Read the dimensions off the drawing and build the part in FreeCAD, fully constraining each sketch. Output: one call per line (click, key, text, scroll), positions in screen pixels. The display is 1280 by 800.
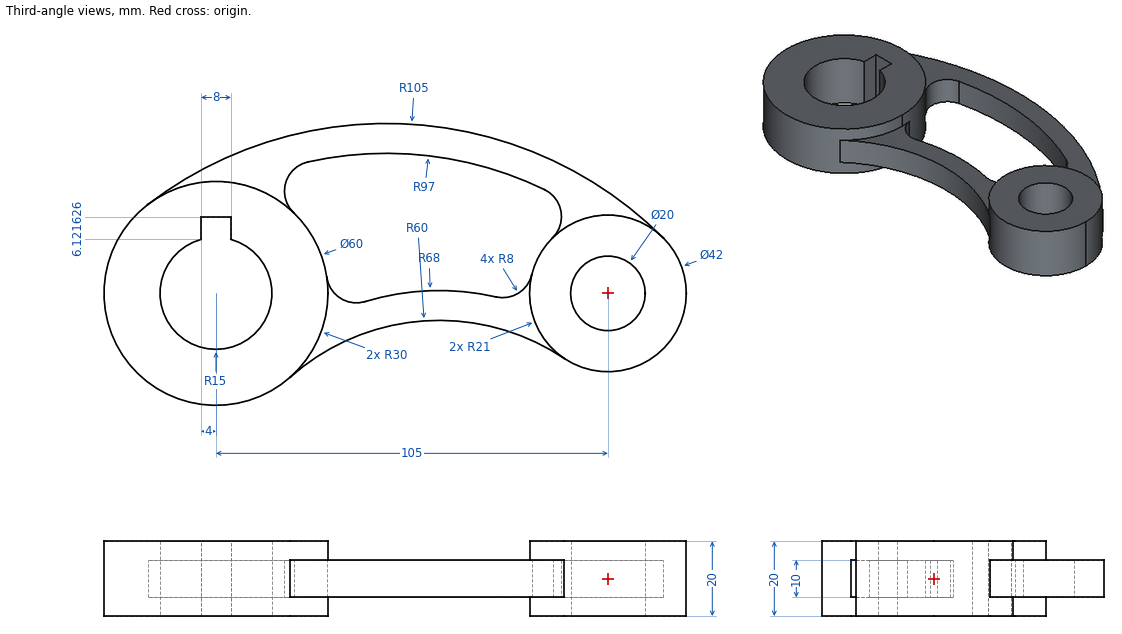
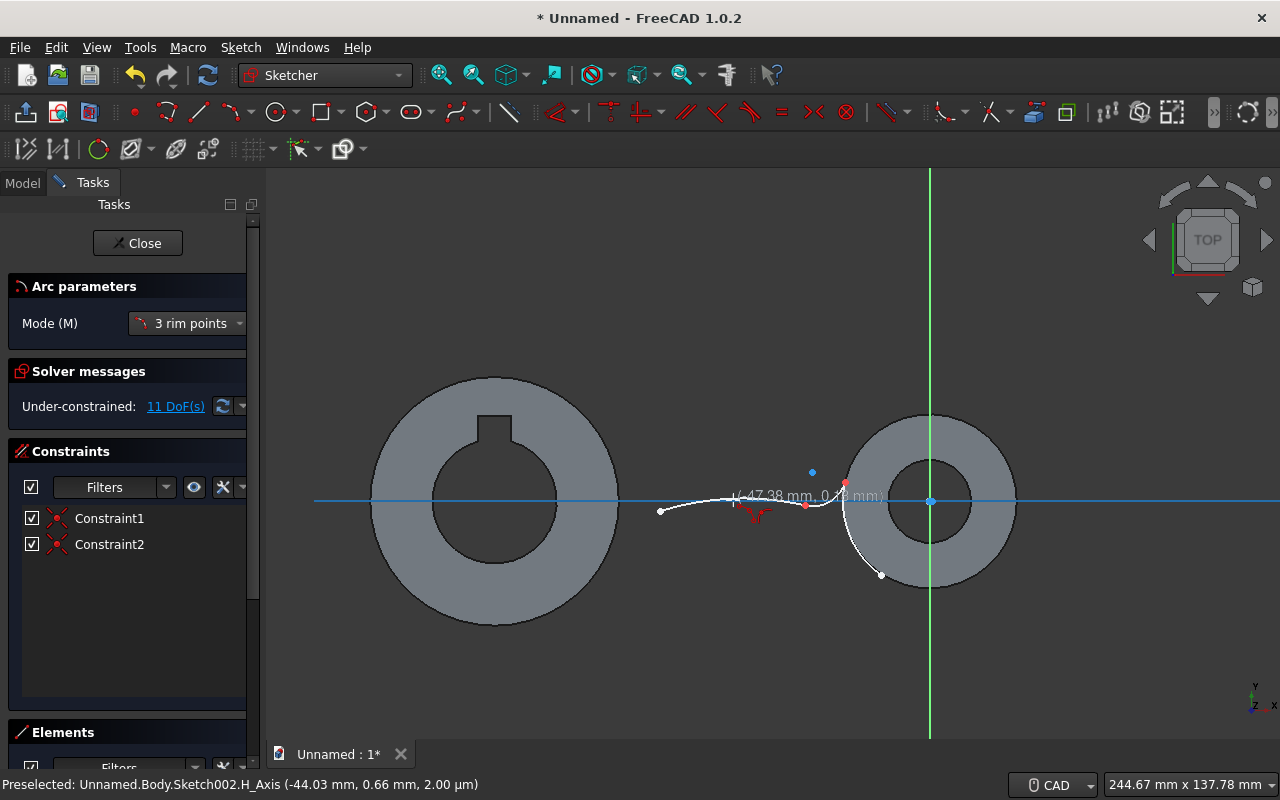
scroll(660, 511, up, 3)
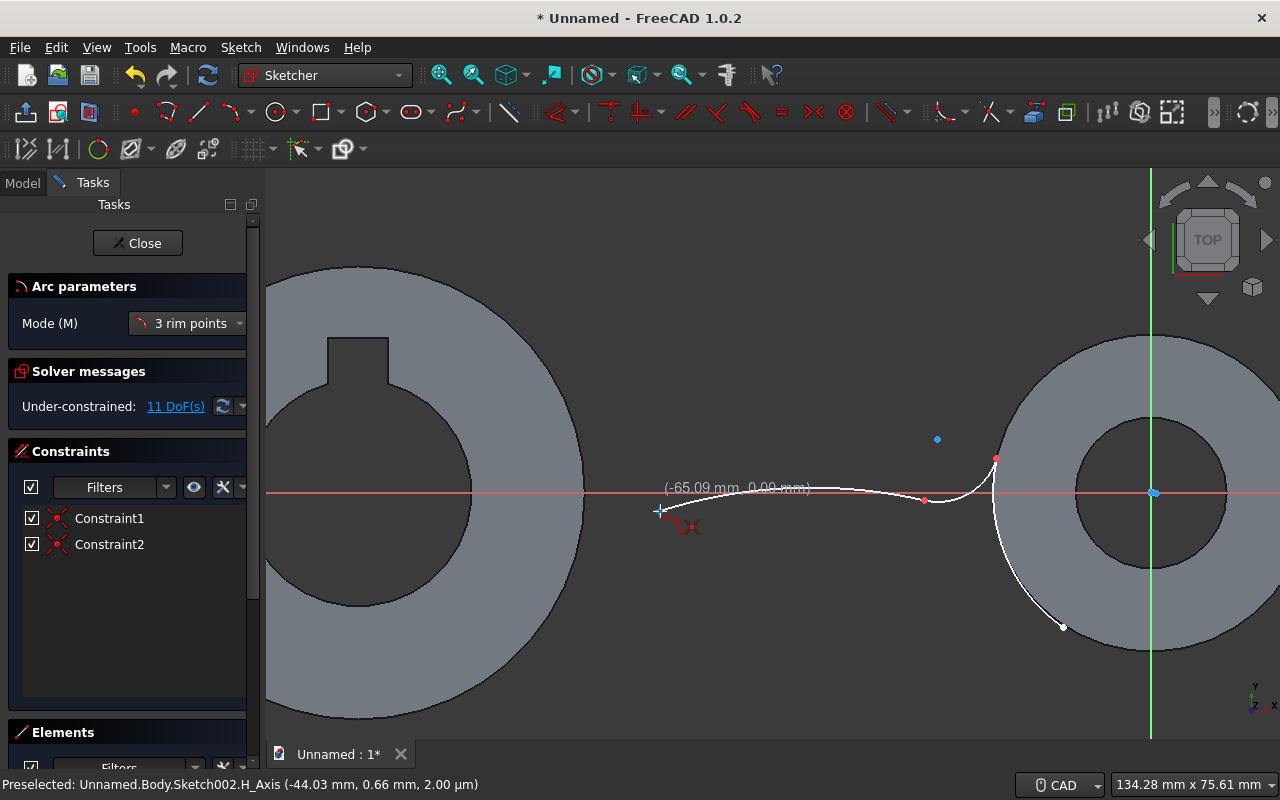
click(660, 511)
click(582, 461)
click(629, 511)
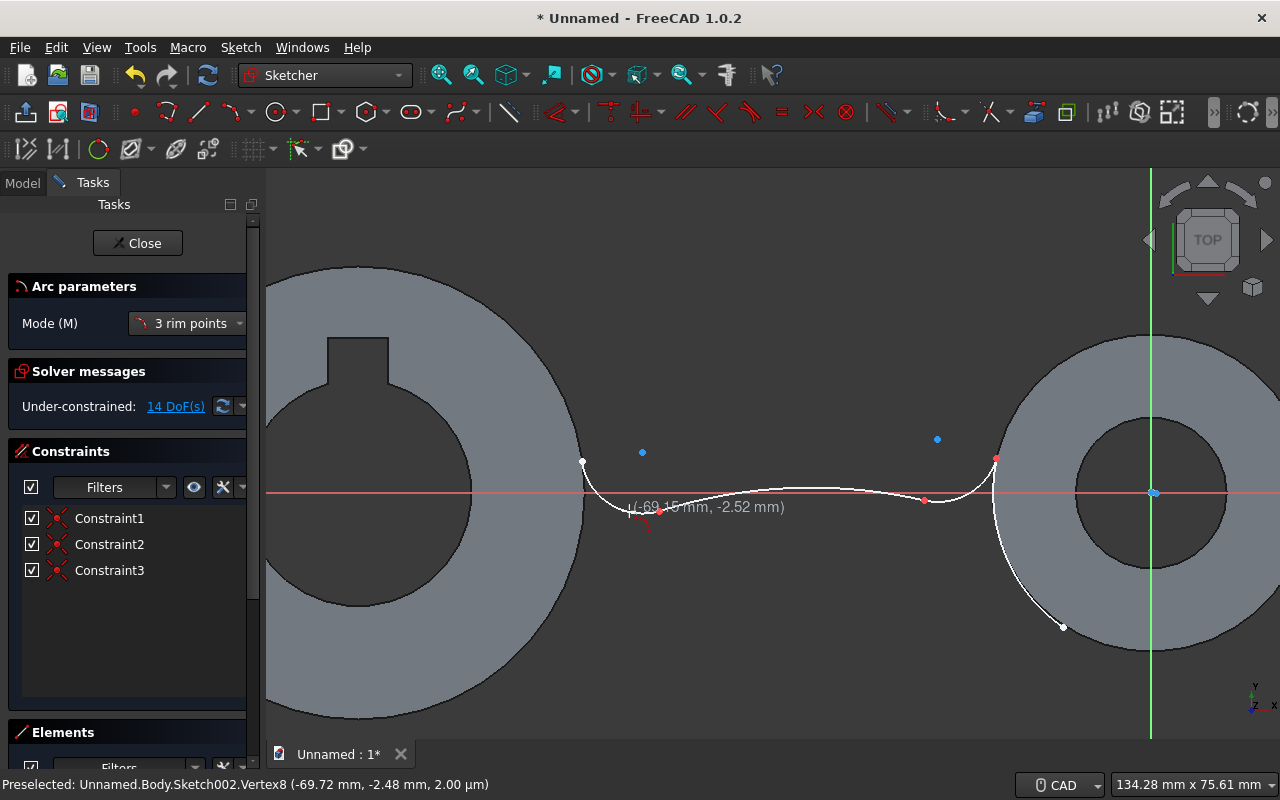
click(582, 462)
click(509, 662)
click(571, 571)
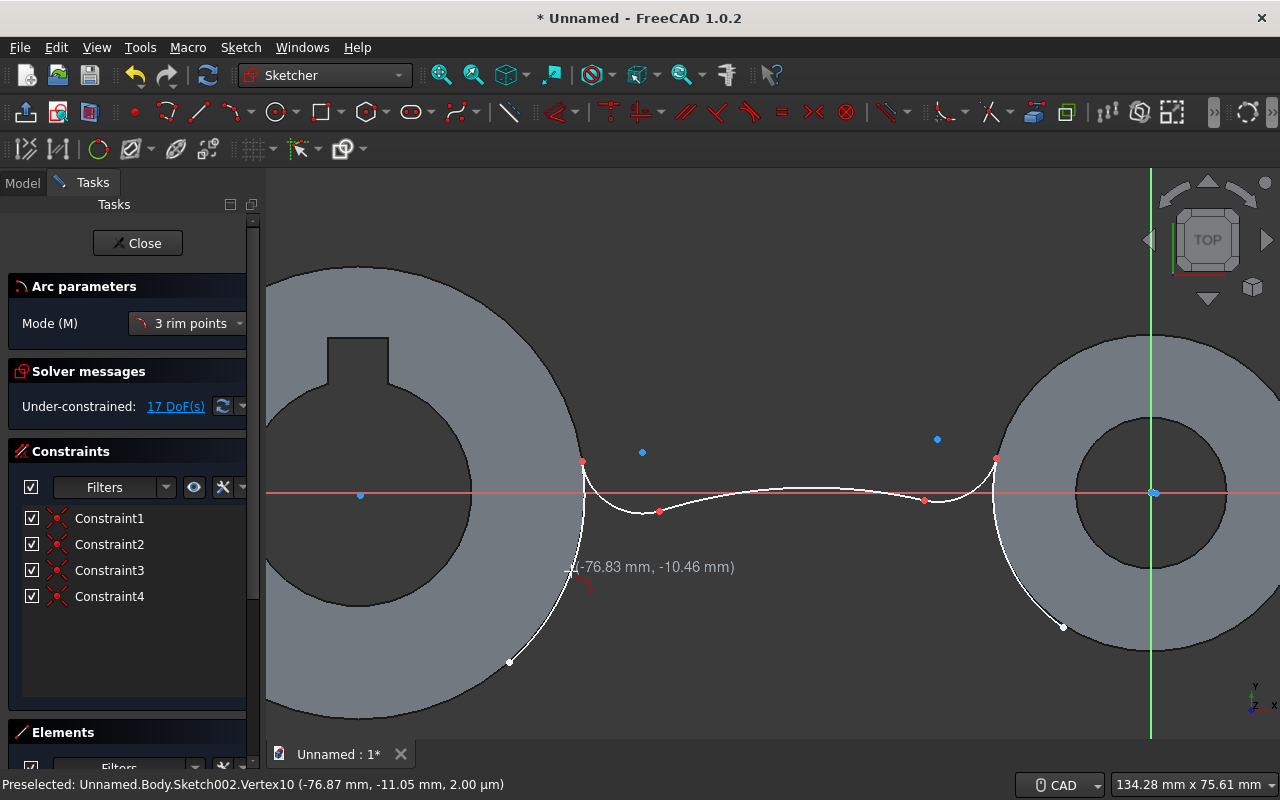
click(509, 663)
click(1064, 628)
click(779, 549)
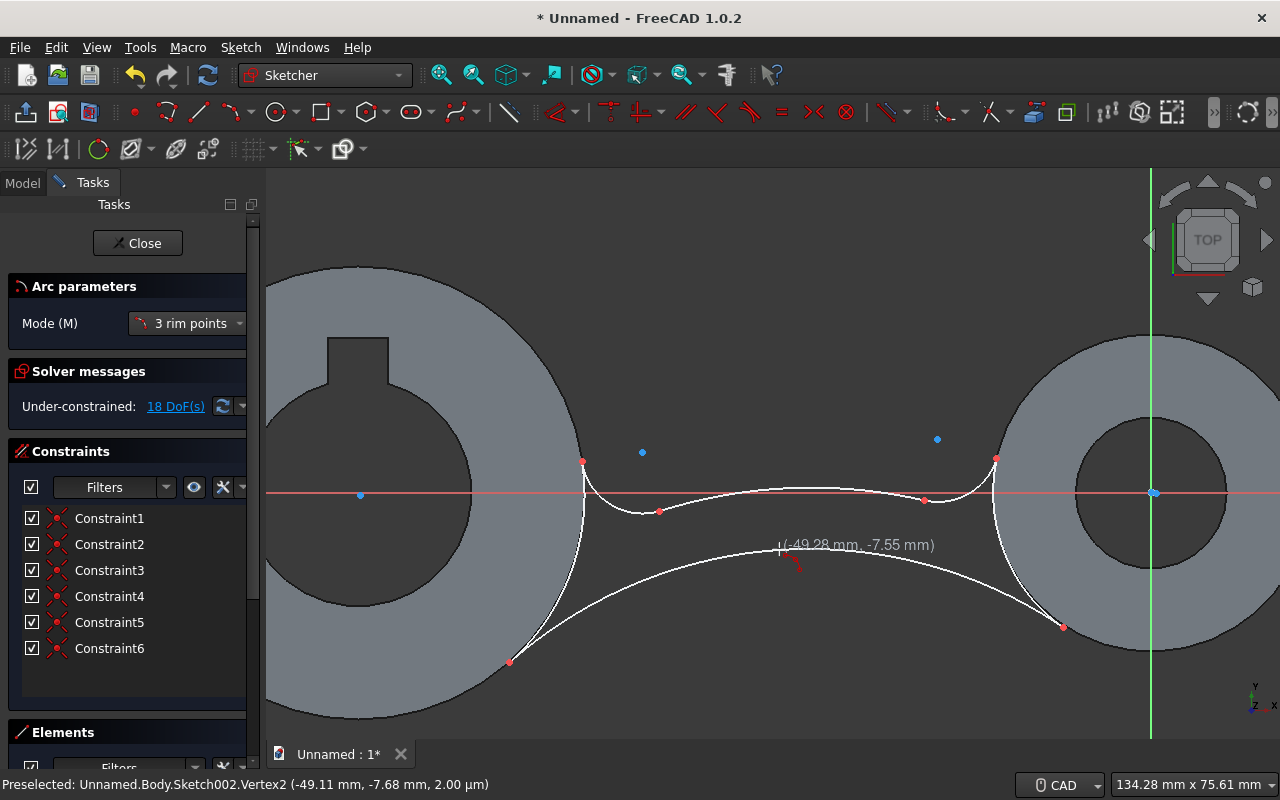
scroll(659, 511, down, 3)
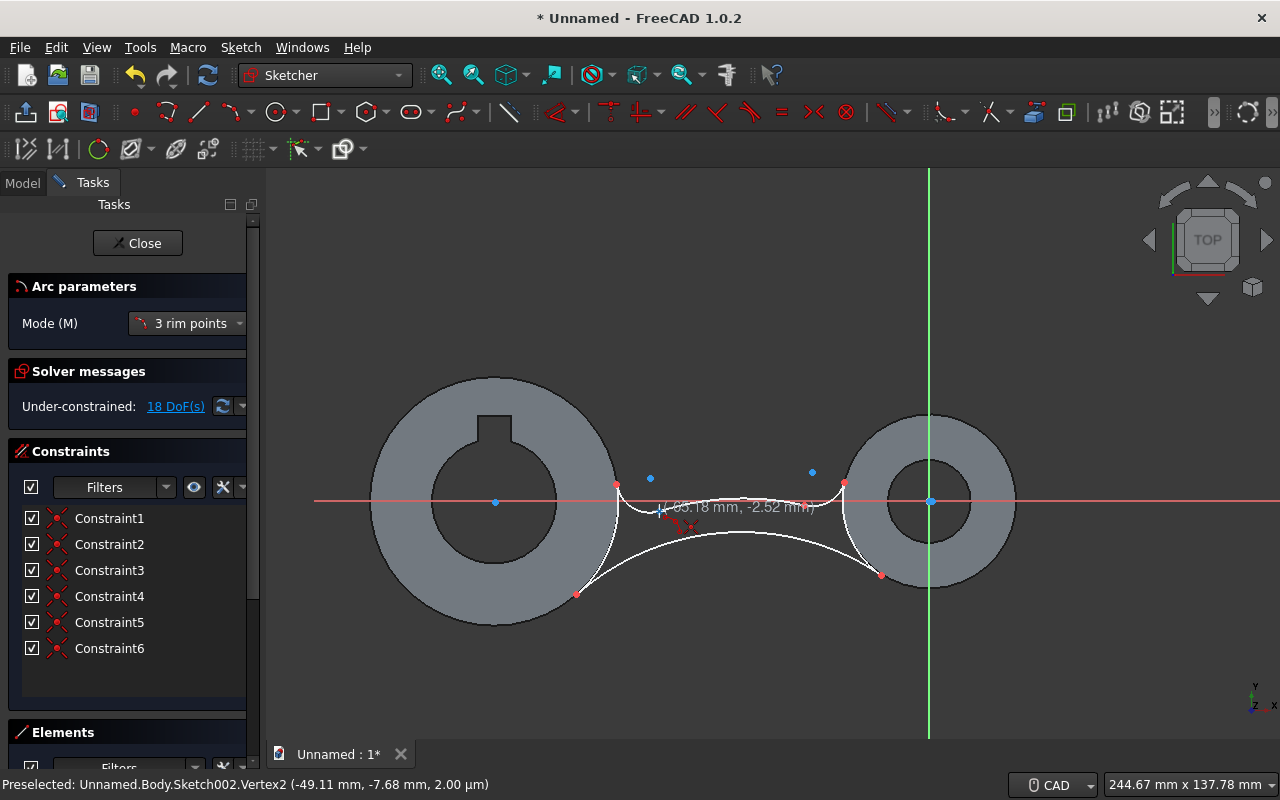
click(991, 440)
click(418, 403)
click(712, 314)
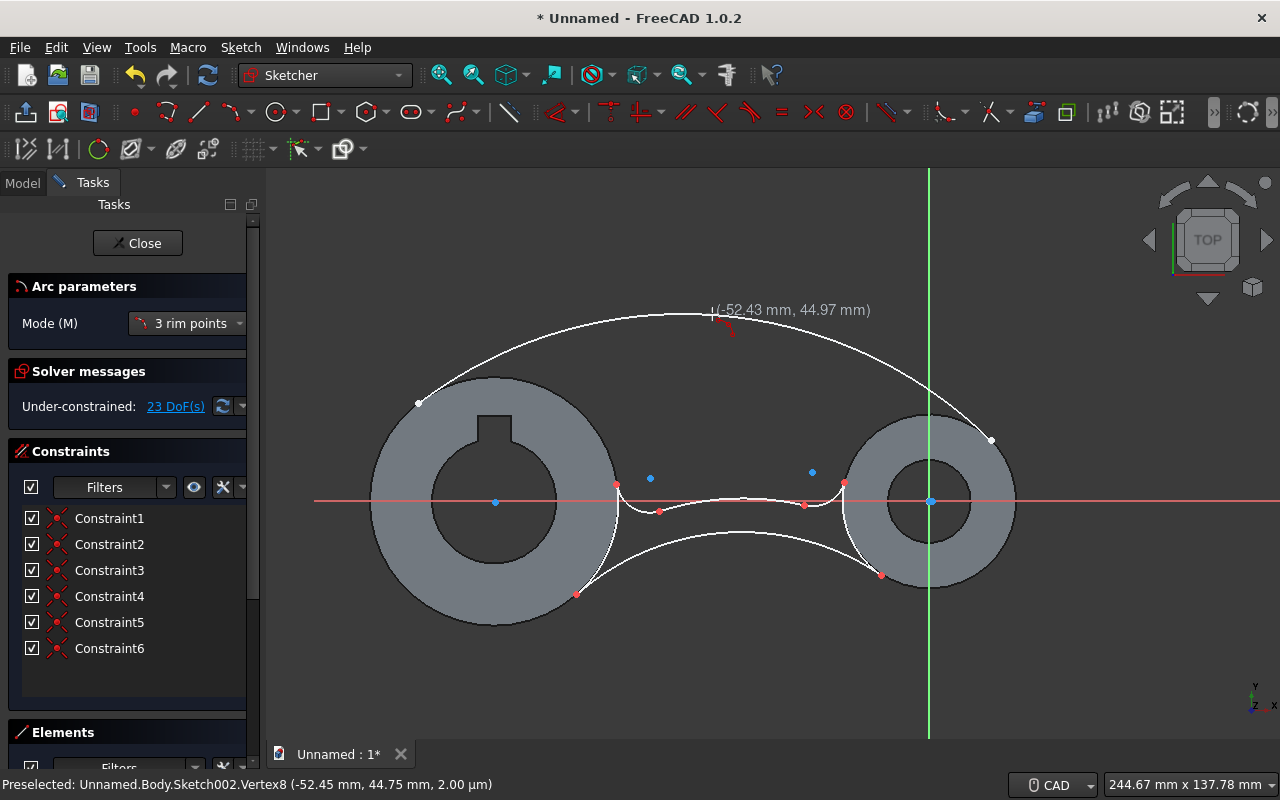
click(418, 404)
click(580, 412)
click(501, 377)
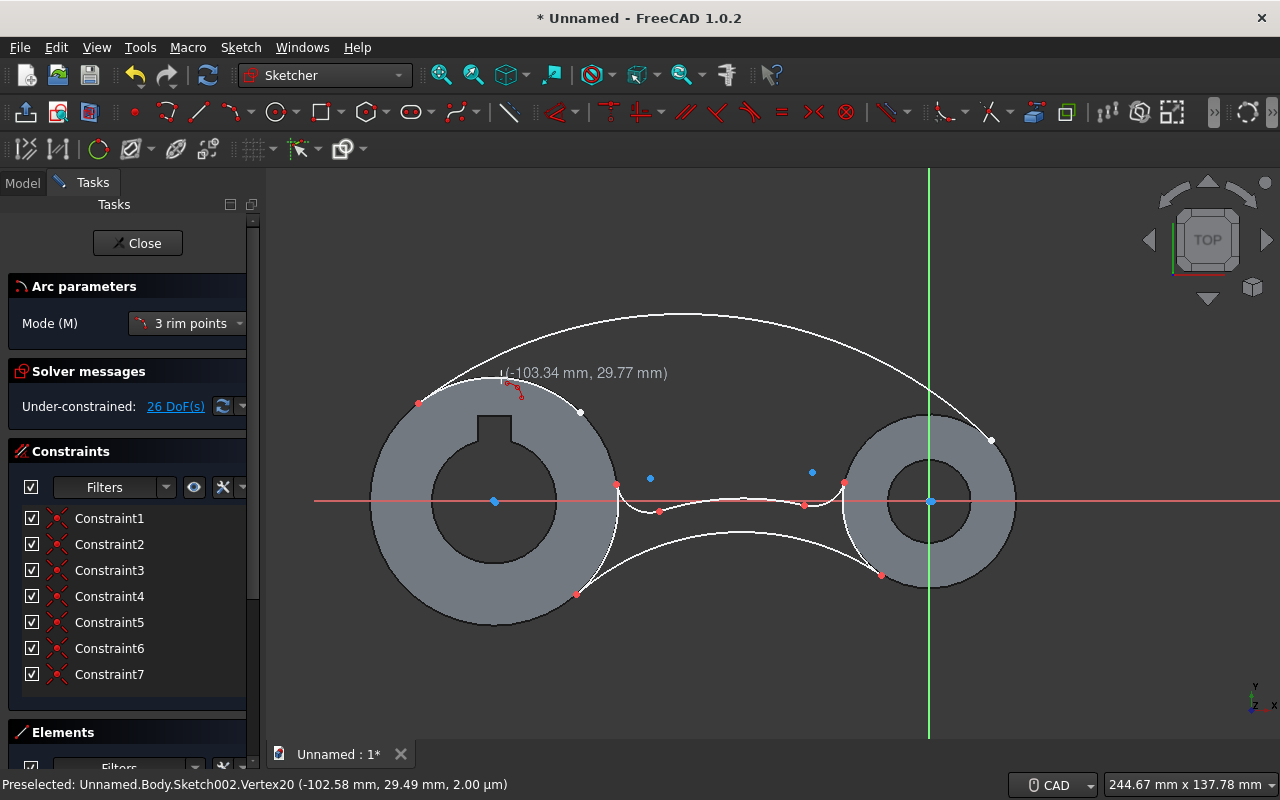
click(580, 413)
click(596, 356)
click(571, 379)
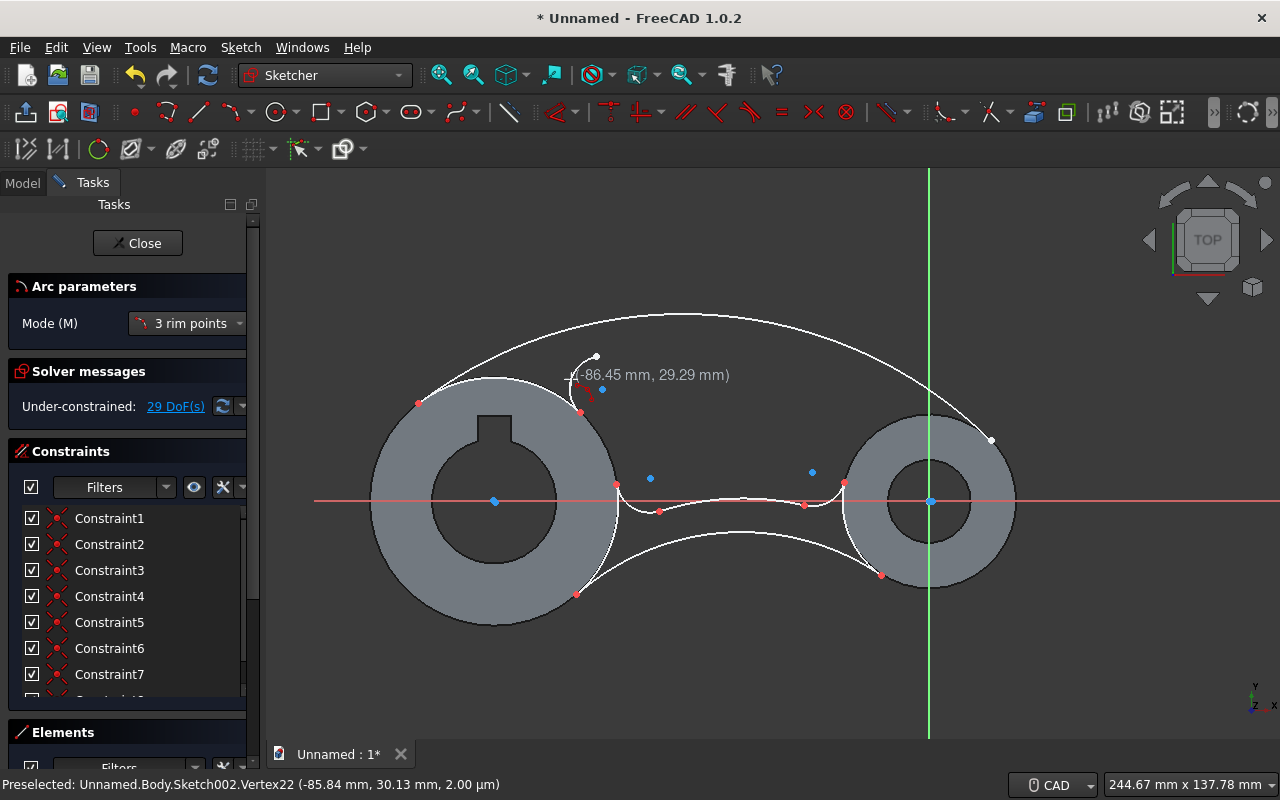
click(596, 357)
click(859, 386)
click(730, 349)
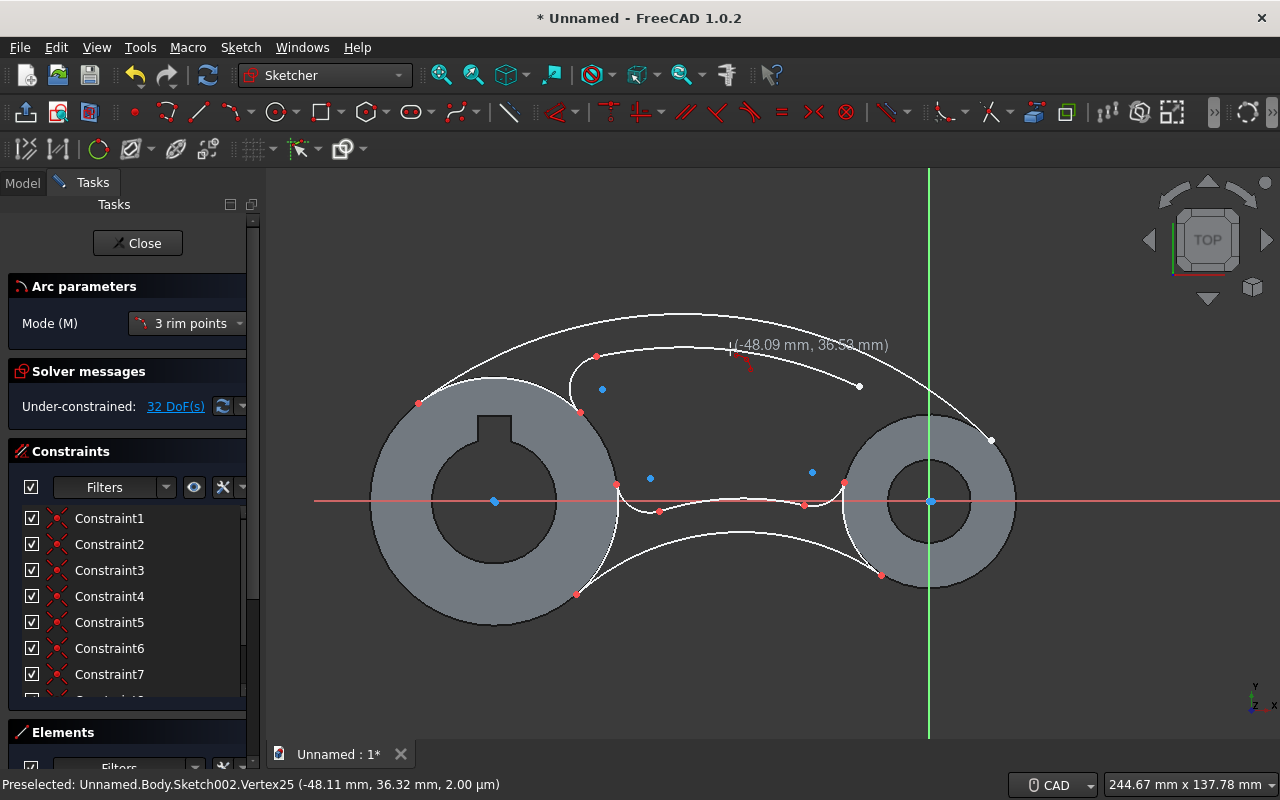
click(859, 387)
click(868, 440)
click(877, 411)